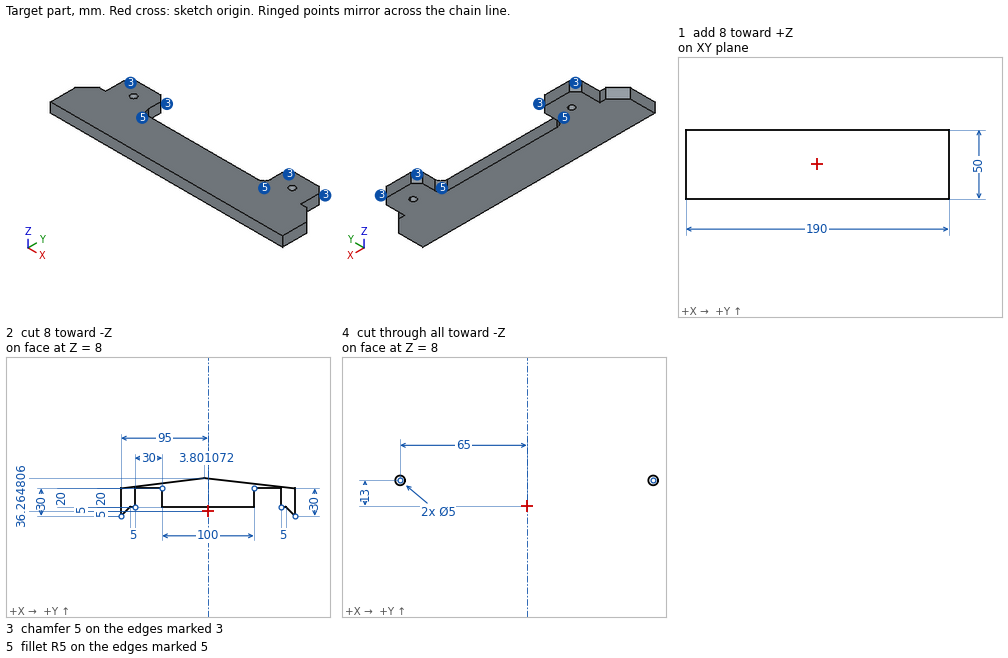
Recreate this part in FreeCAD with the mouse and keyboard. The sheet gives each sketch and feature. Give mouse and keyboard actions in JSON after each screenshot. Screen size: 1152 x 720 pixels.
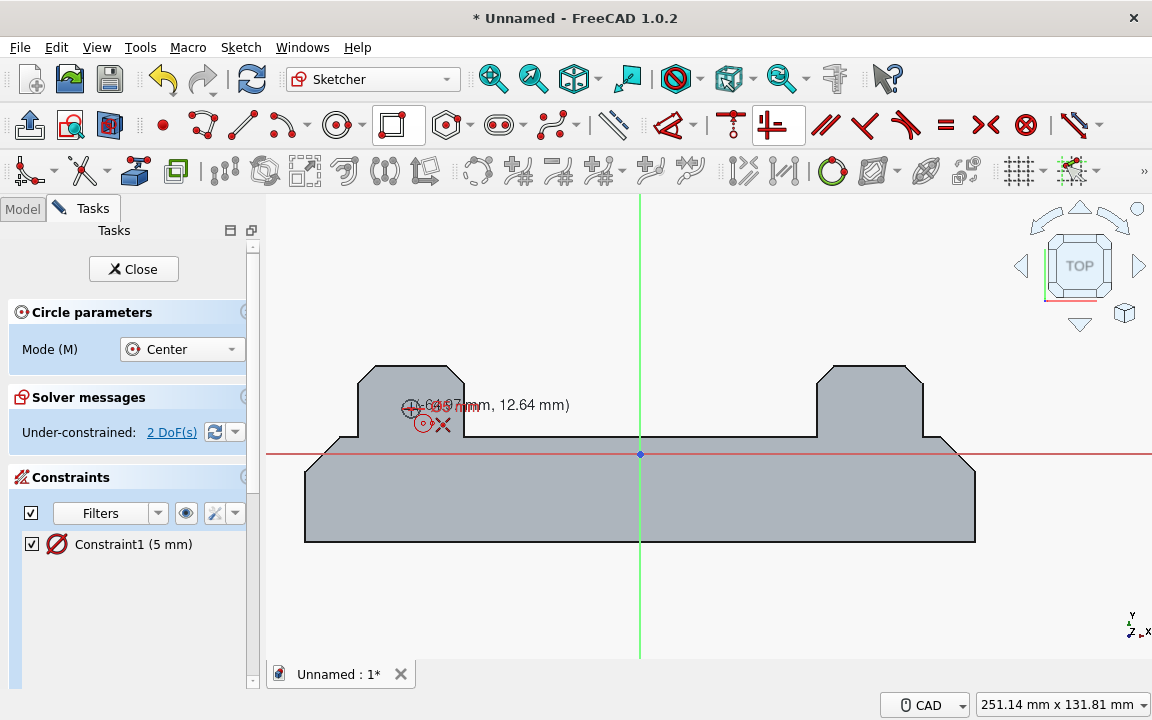
{"action": "scroll", "coordinate": [870, 408], "scroll_direction": "up", "scroll_amount": 5}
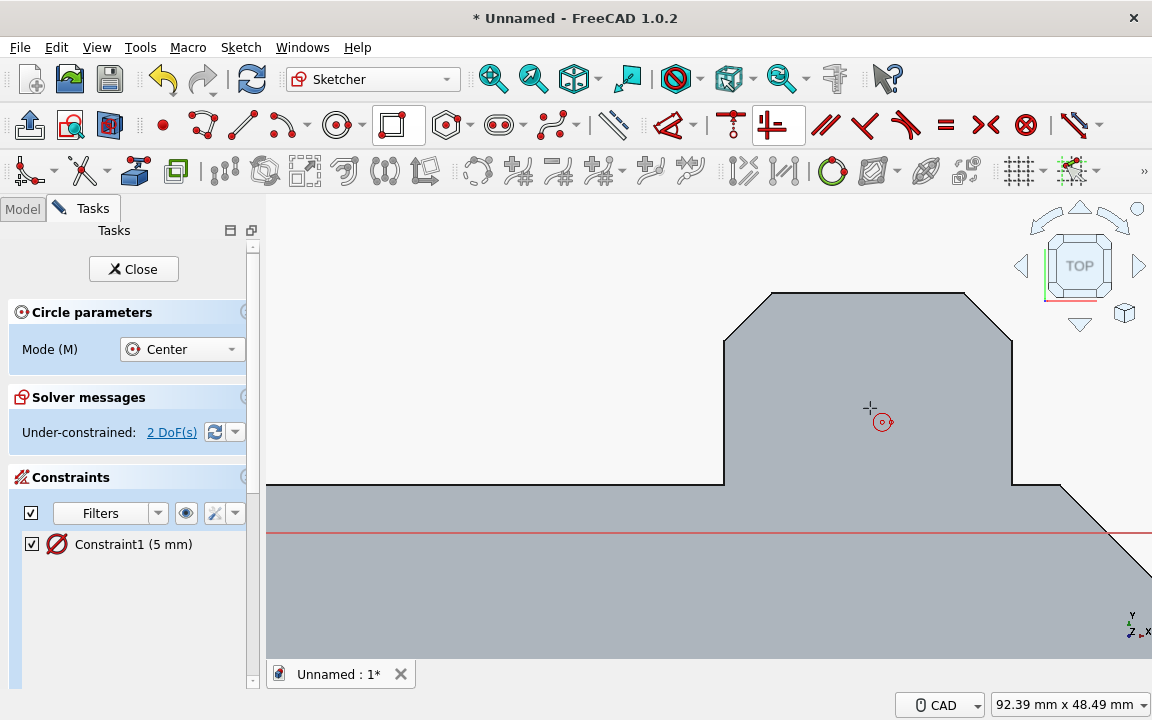
{"action": "left_click", "coordinate": [868, 408]}
{"action": "mouse_move", "coordinate": [885, 391]}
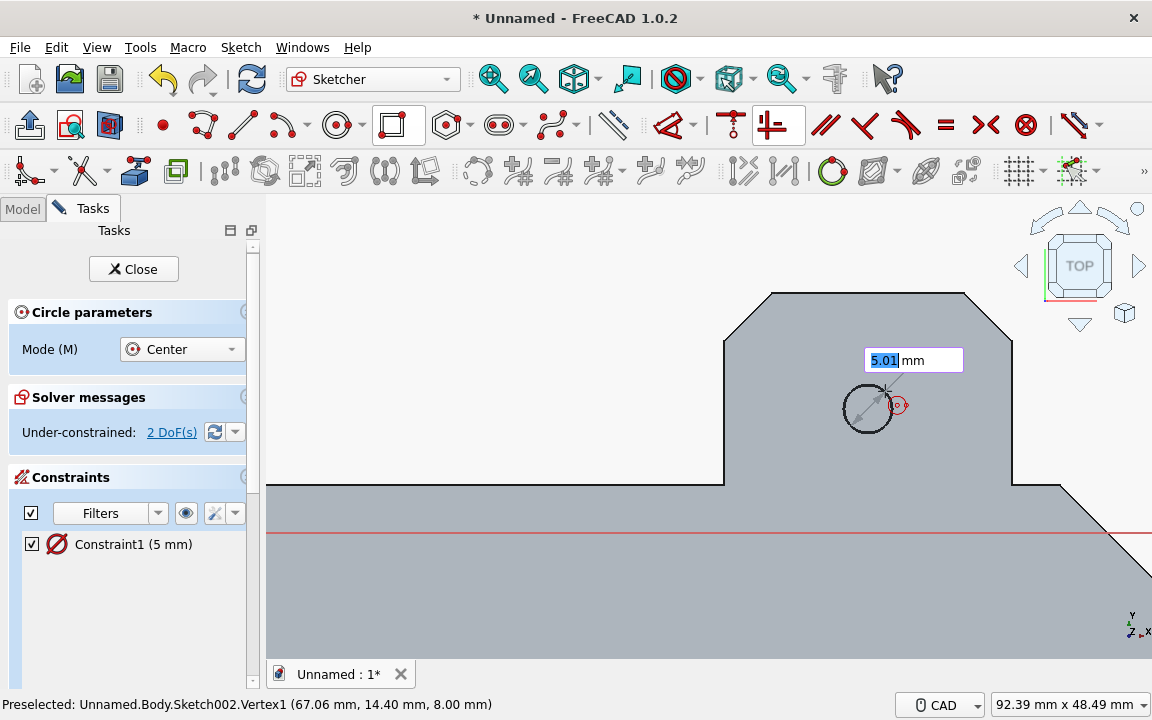
{"action": "type", "text": "5"}
{"action": "key", "text": "Return"}
{"action": "key", "text": "Escape"}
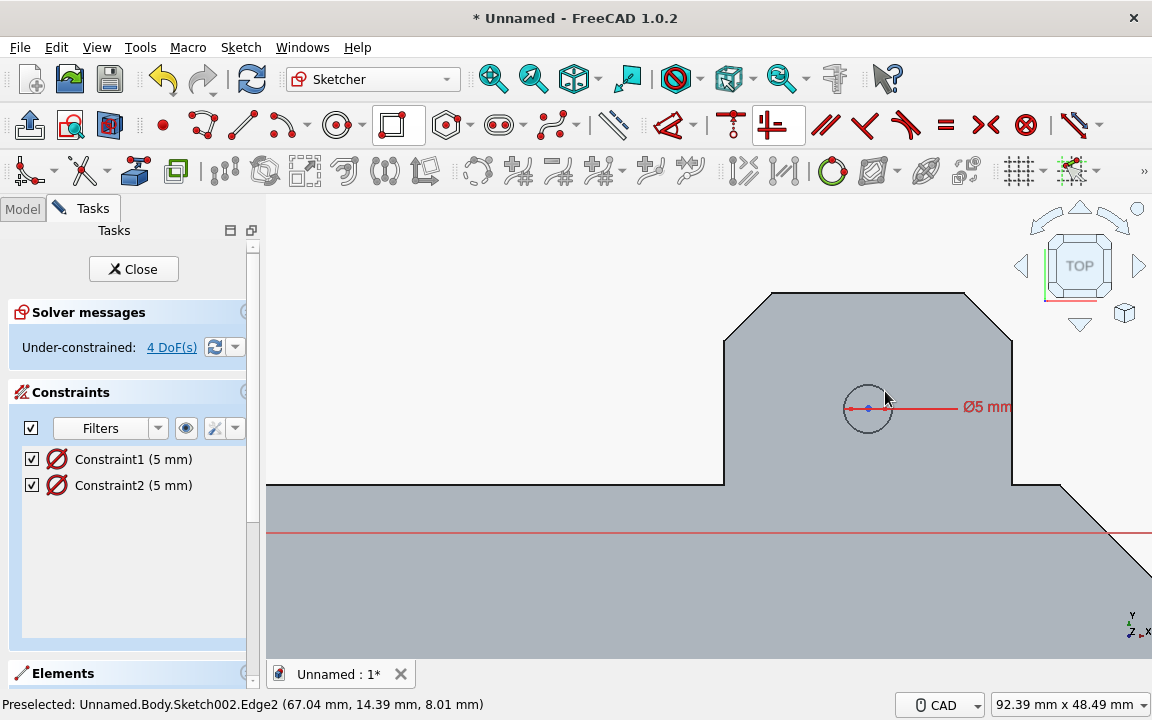
{"action": "scroll", "coordinate": [871, 408], "scroll_direction": "down", "scroll_amount": 5}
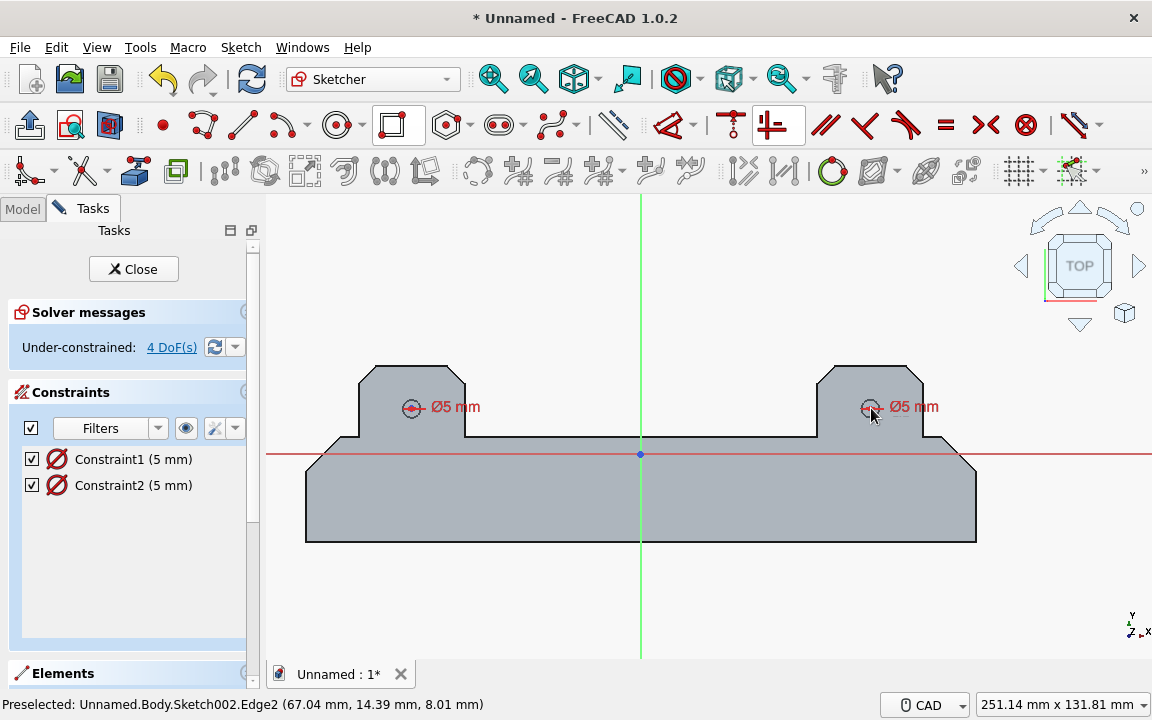
{"action": "left_click", "coordinate": [412, 409]}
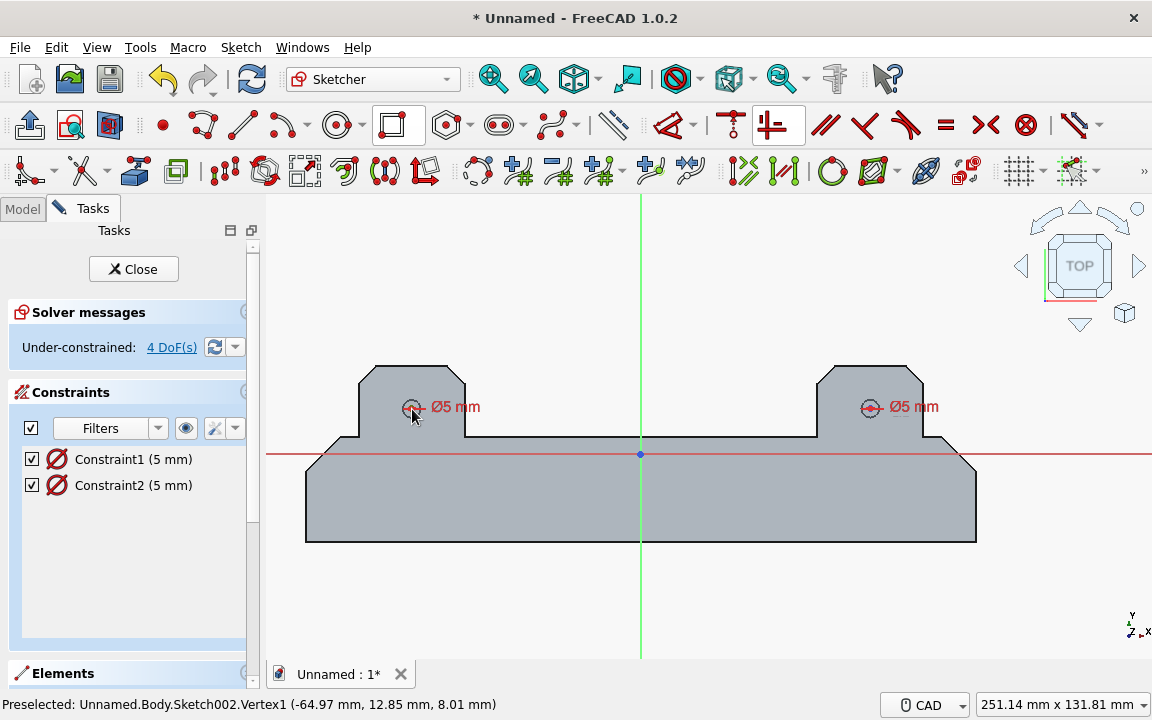
{"action": "left_click", "coordinate": [870, 409]}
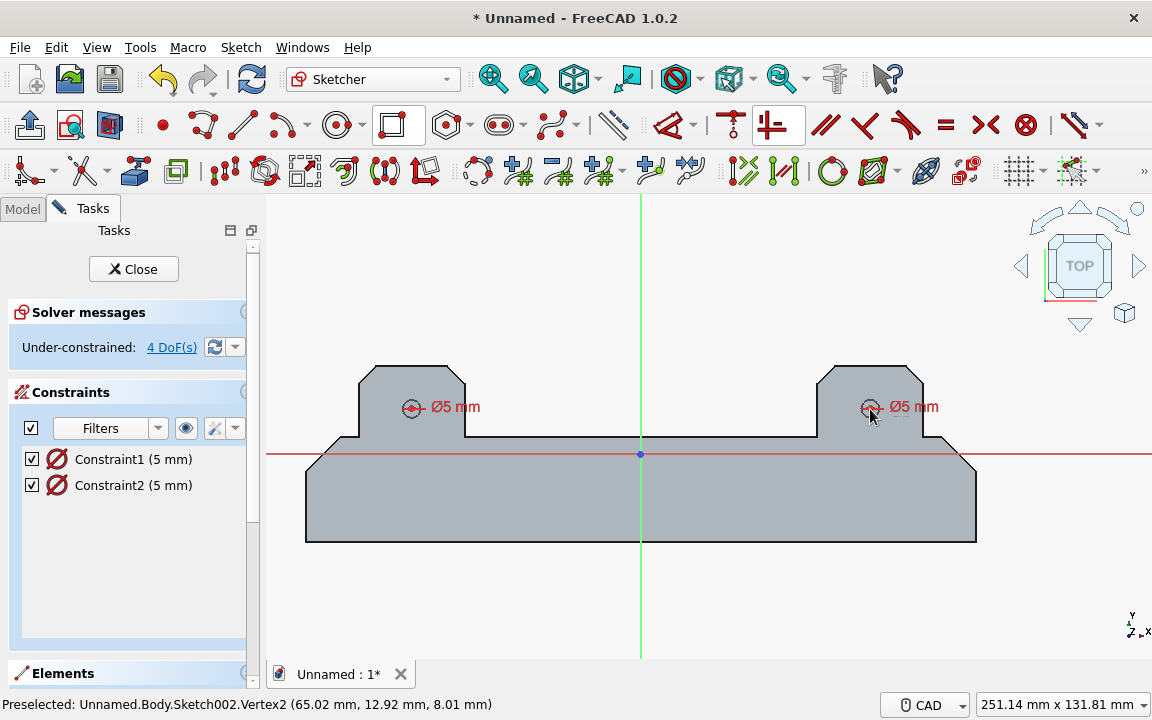
{"action": "left_click", "coordinate": [641, 602]}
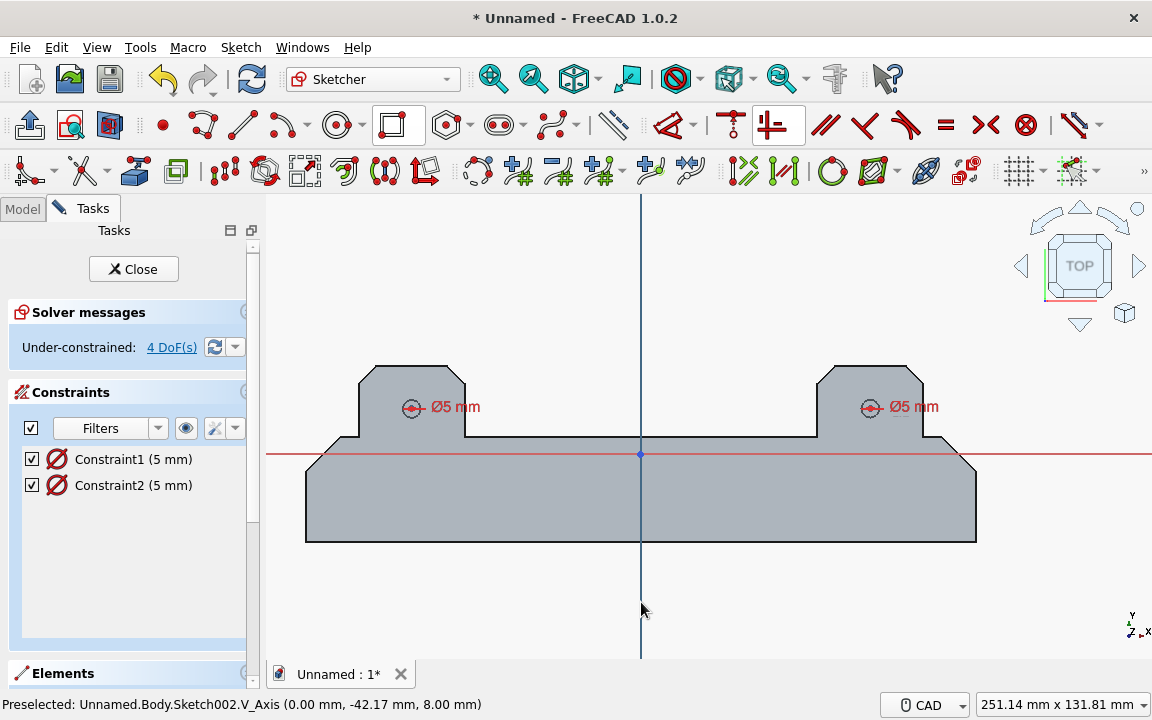
{"action": "left_click", "coordinate": [986, 126]}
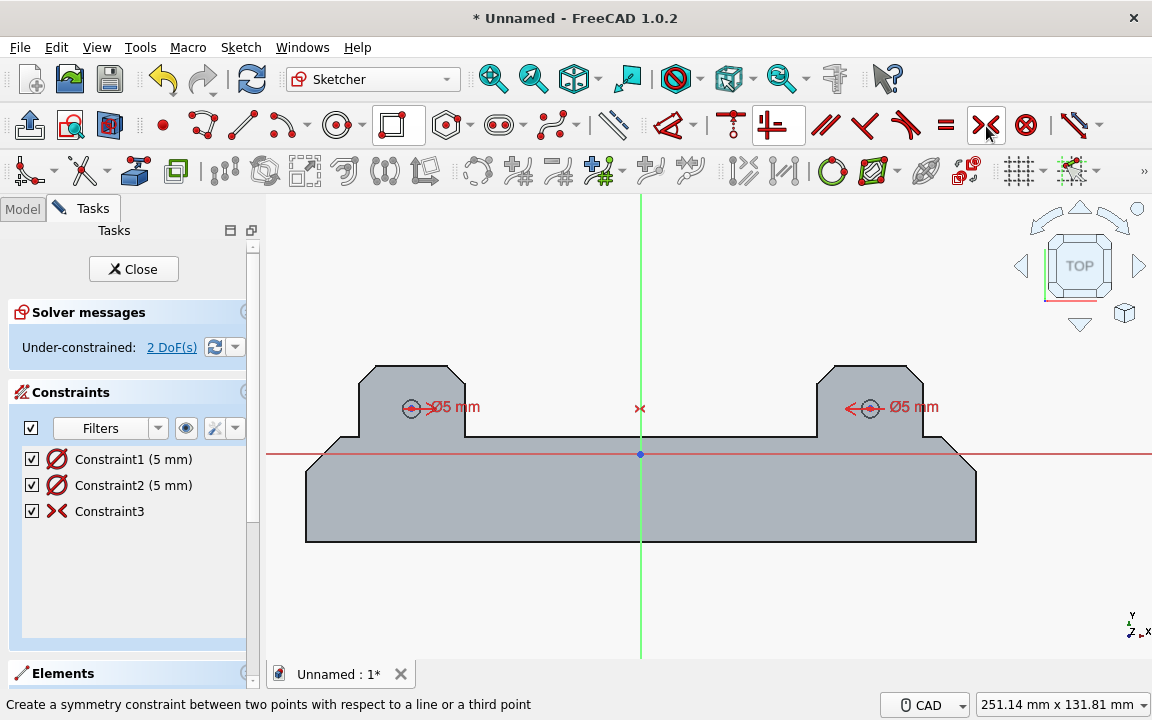
{"action": "left_click", "coordinate": [668, 126]}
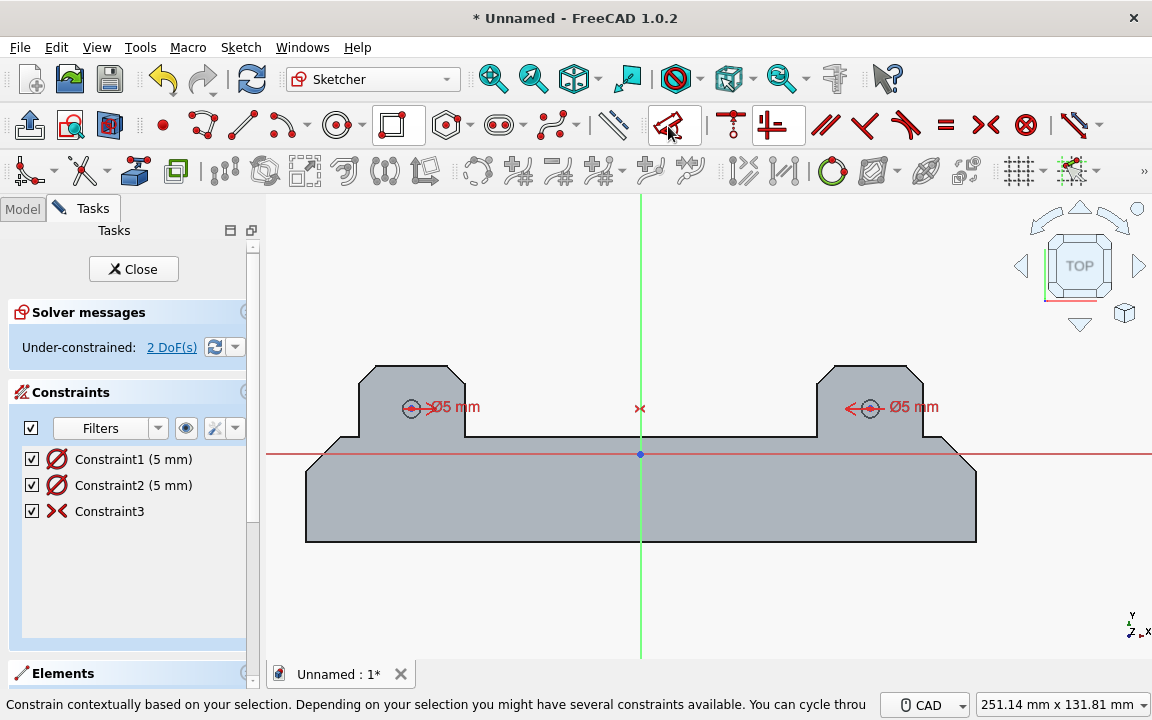
{"action": "left_click", "coordinate": [412, 409]}
{"action": "left_click", "coordinate": [526, 488]}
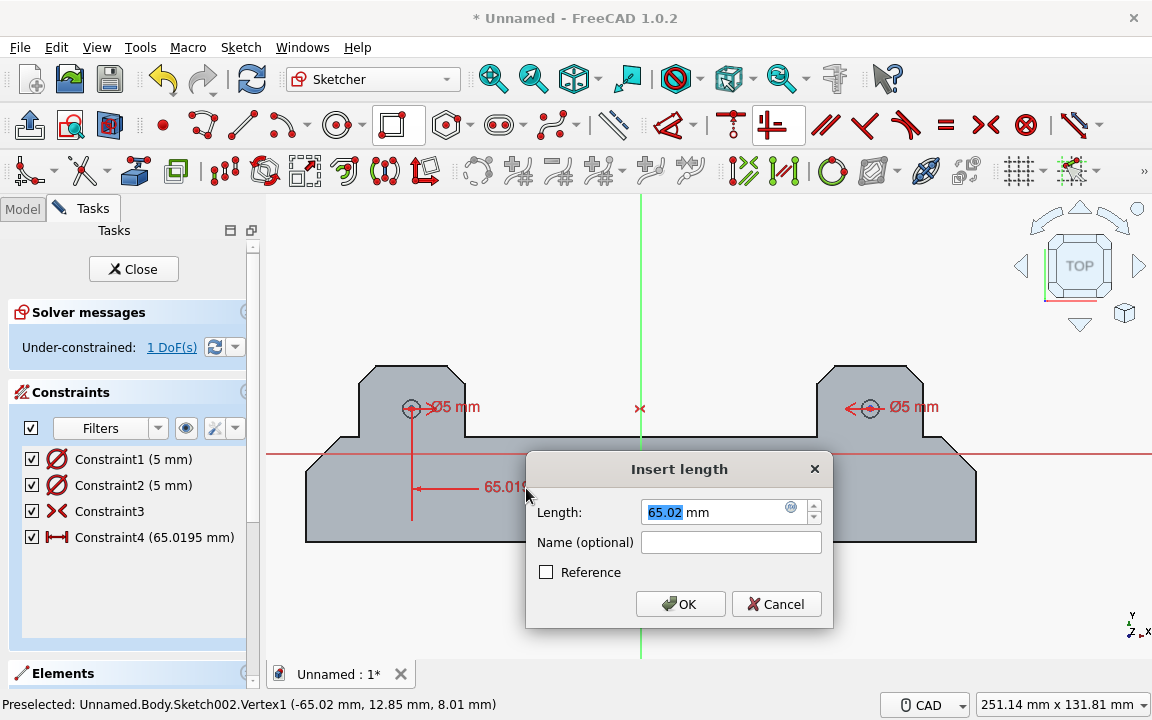
{"action": "type", "text": "65"}
{"action": "key", "text": "Return"}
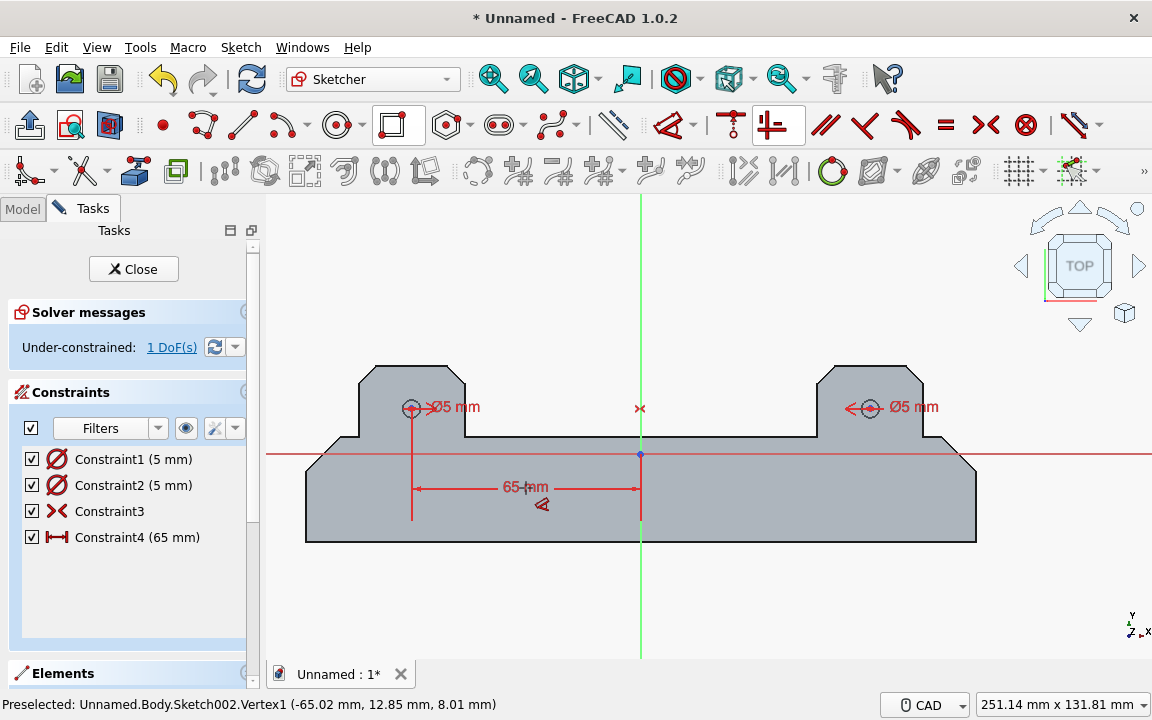
{"action": "left_click", "coordinate": [412, 409]}
{"action": "left_click", "coordinate": [378, 432]}